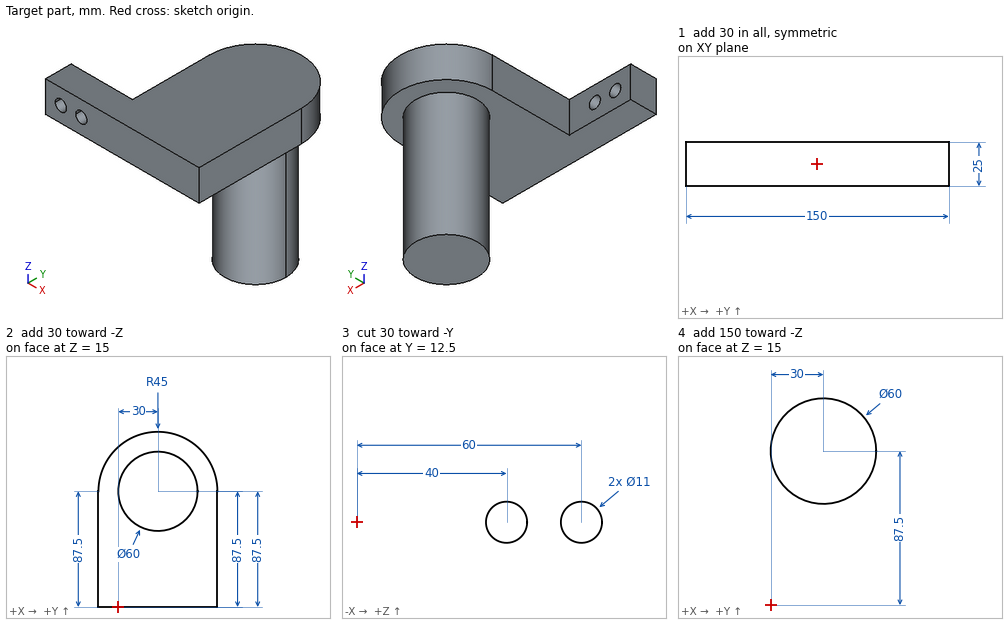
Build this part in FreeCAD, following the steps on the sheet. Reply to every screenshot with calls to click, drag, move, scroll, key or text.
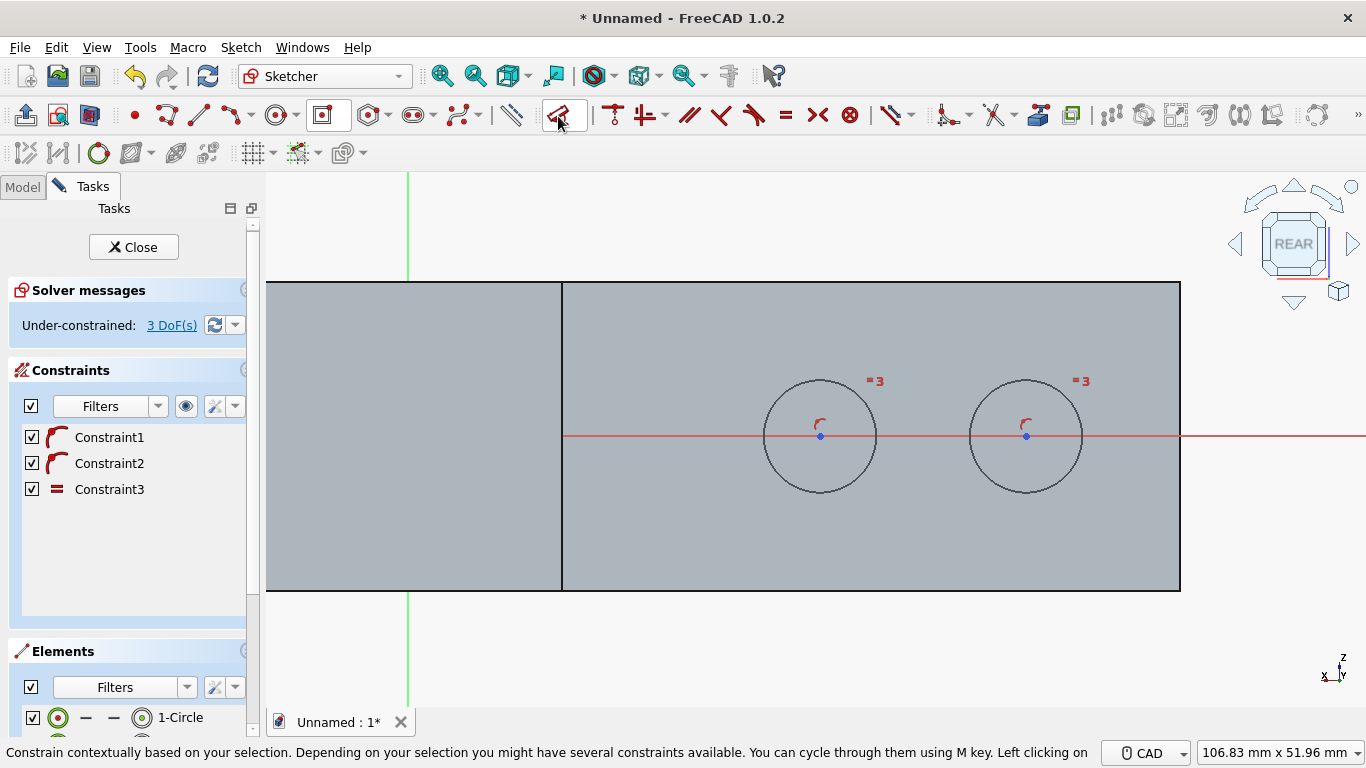
click(1066, 397)
click(1089, 375)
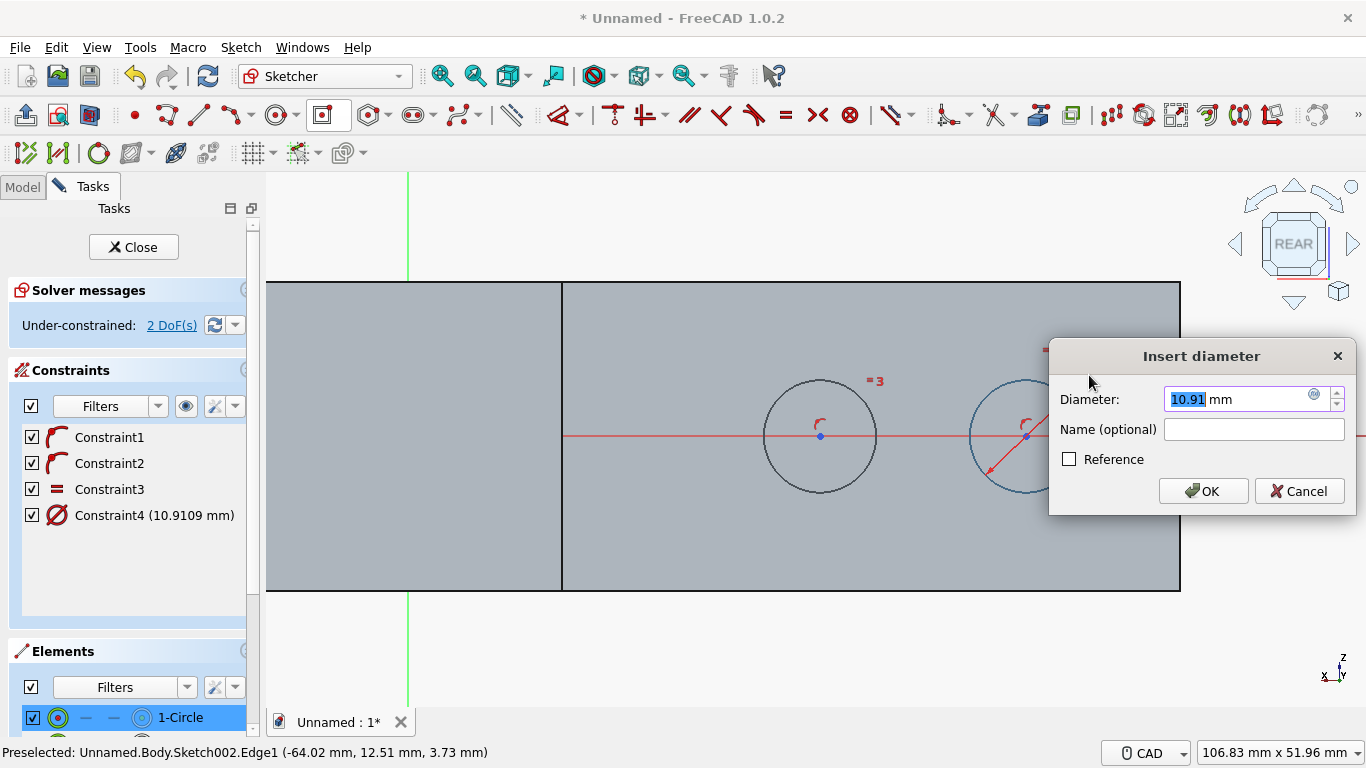
text(11)
key(Return)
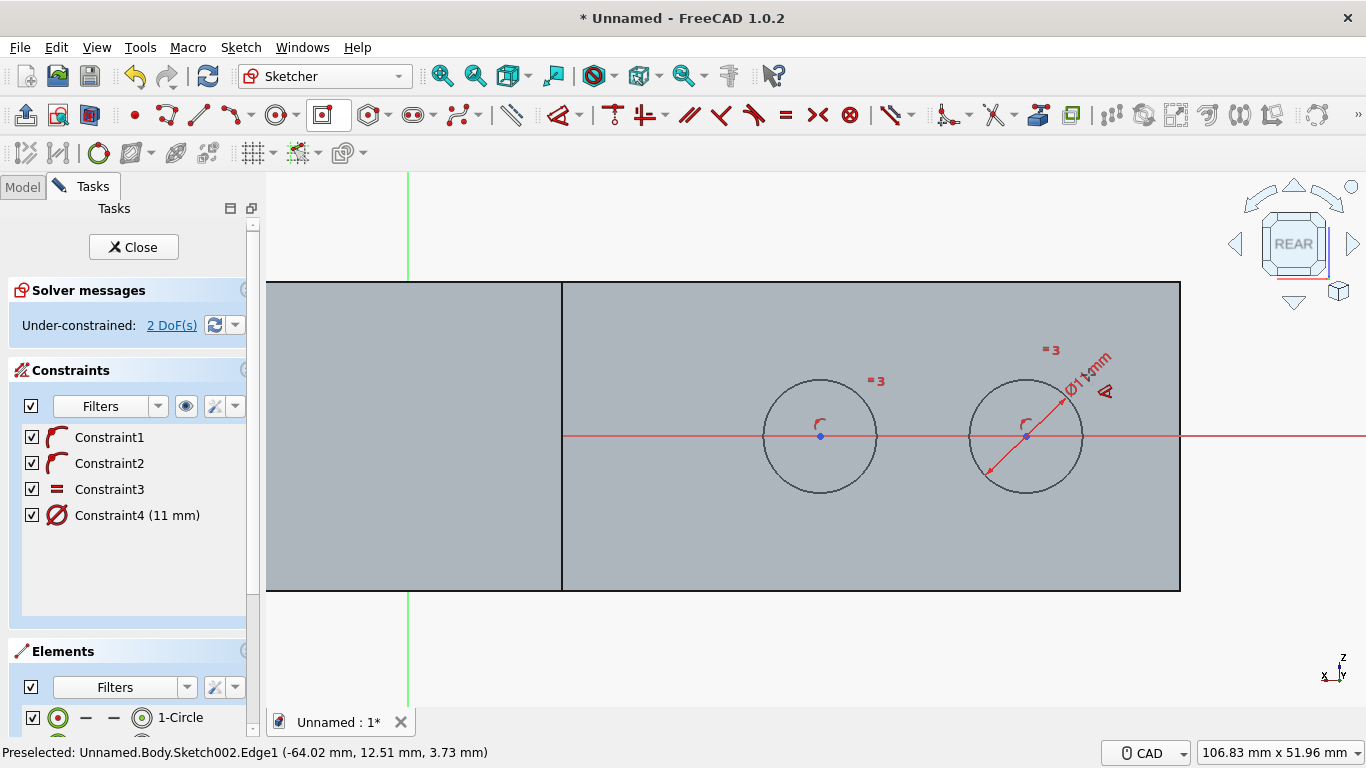
click(1026, 436)
click(717, 470)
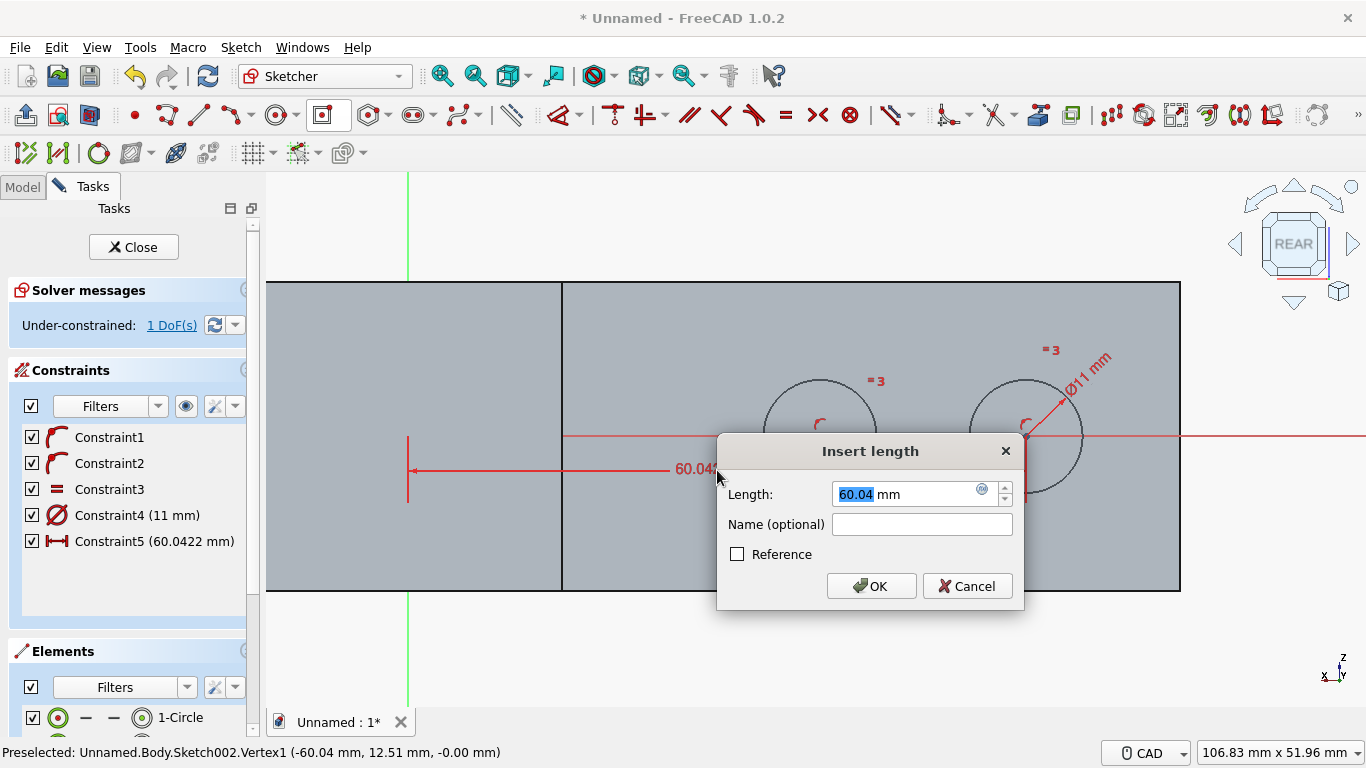
text(60)
key(Return)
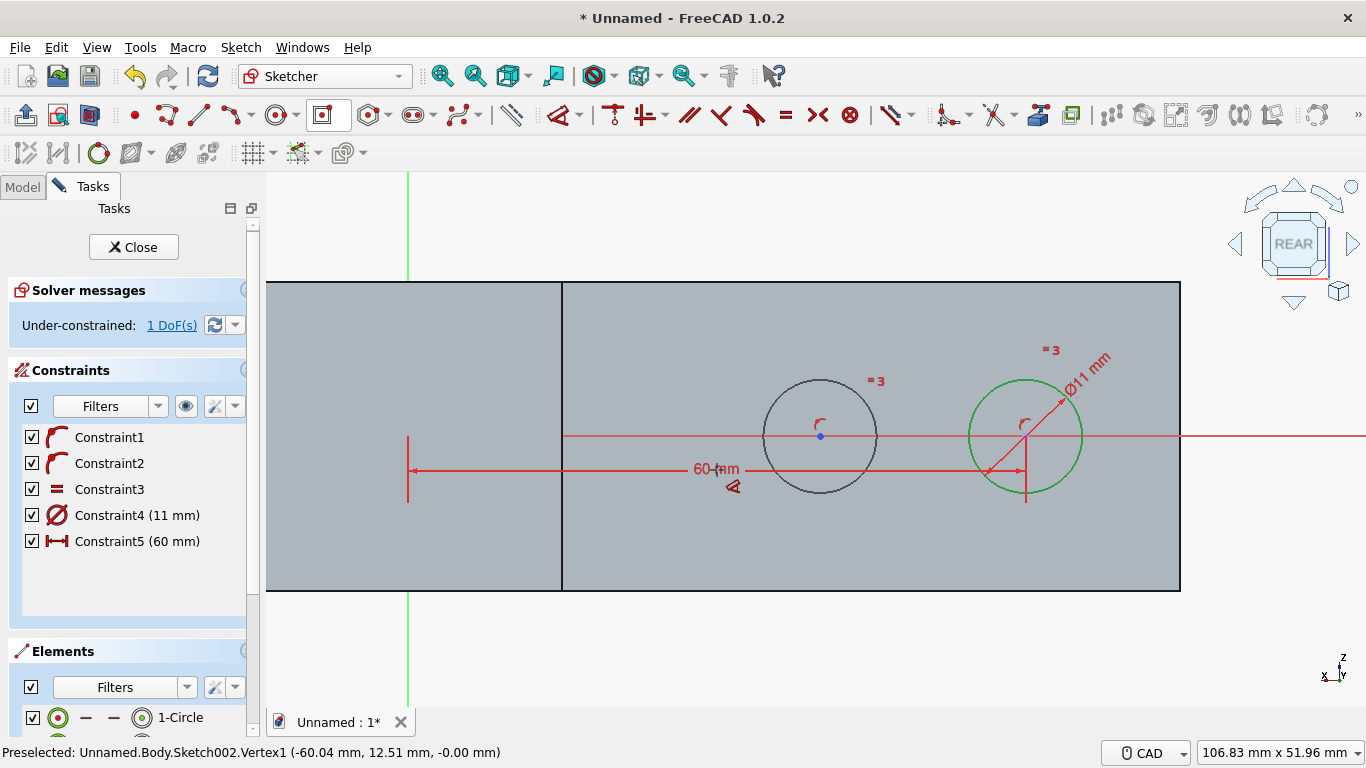
click(820, 436)
click(614, 470)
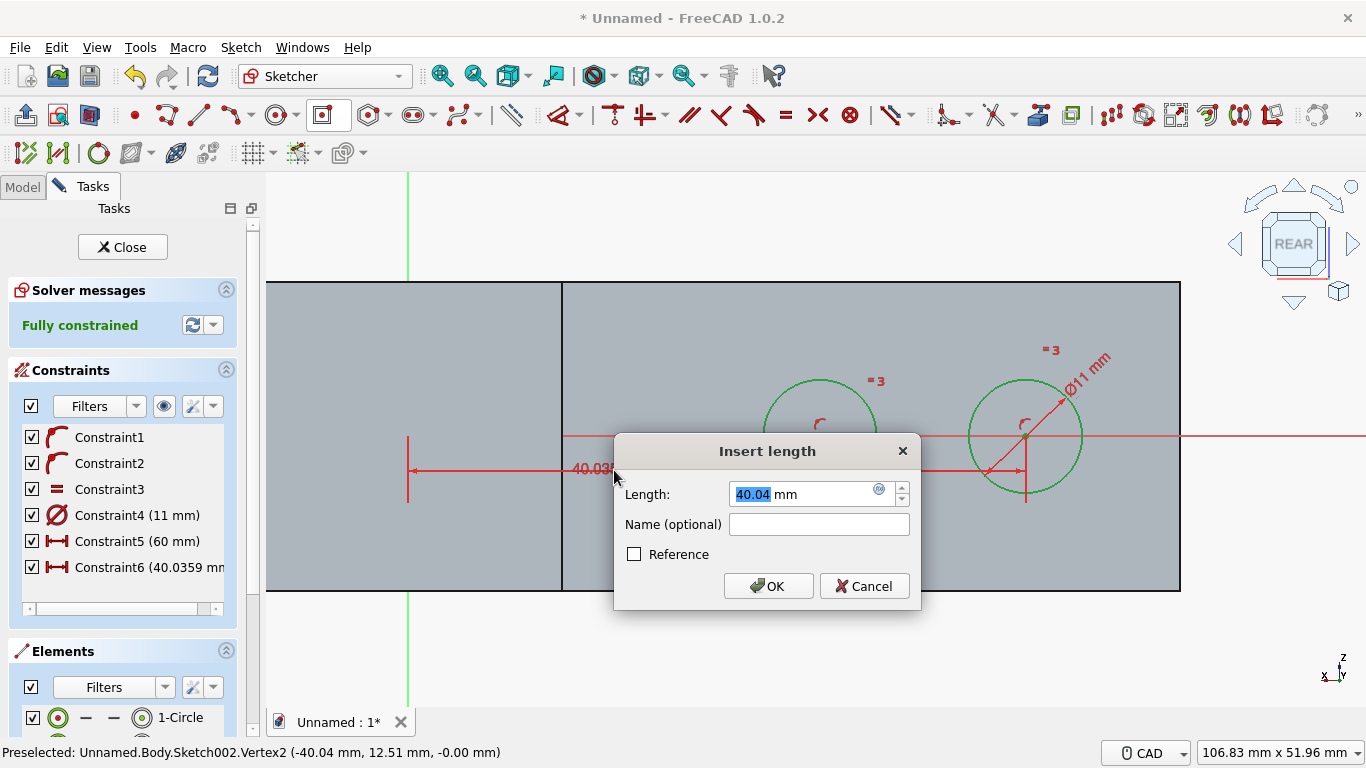
text(40)
key(Return)
key(Escape)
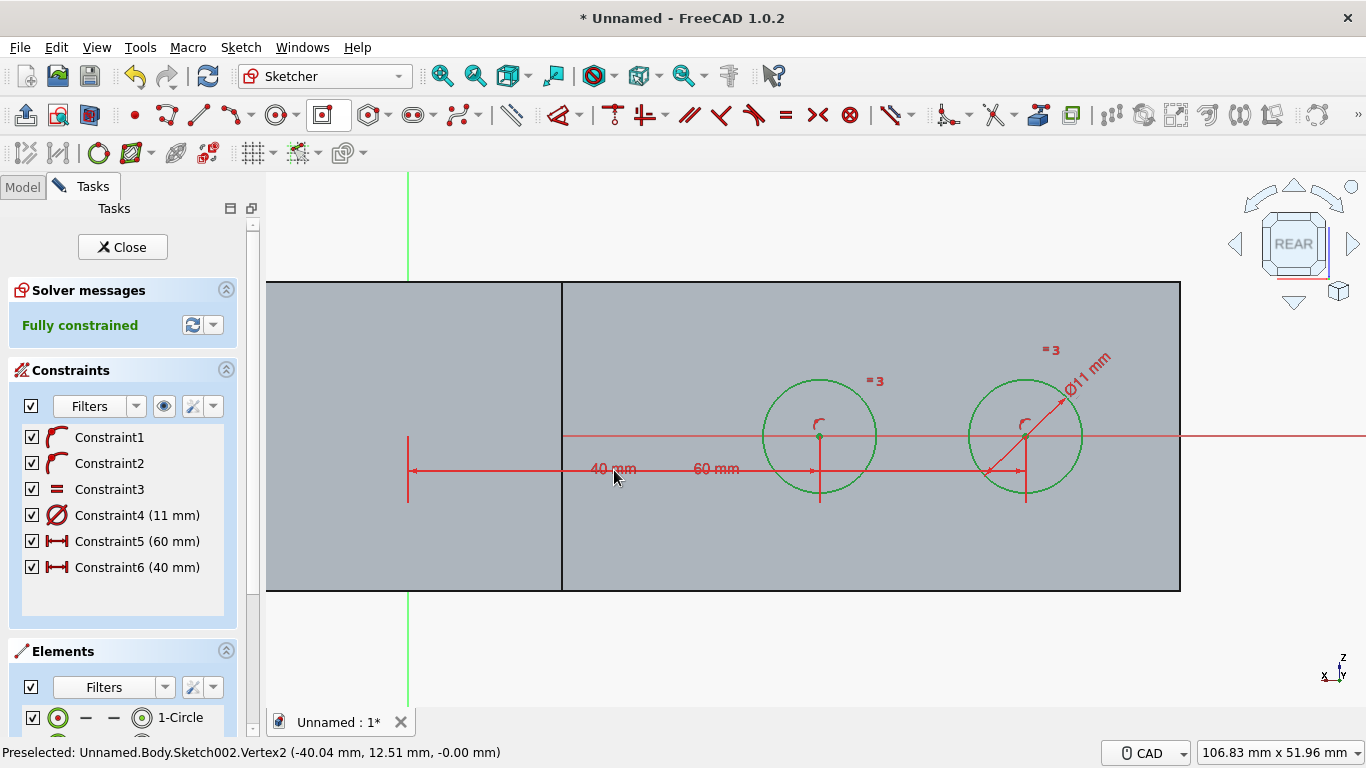
click(123, 247)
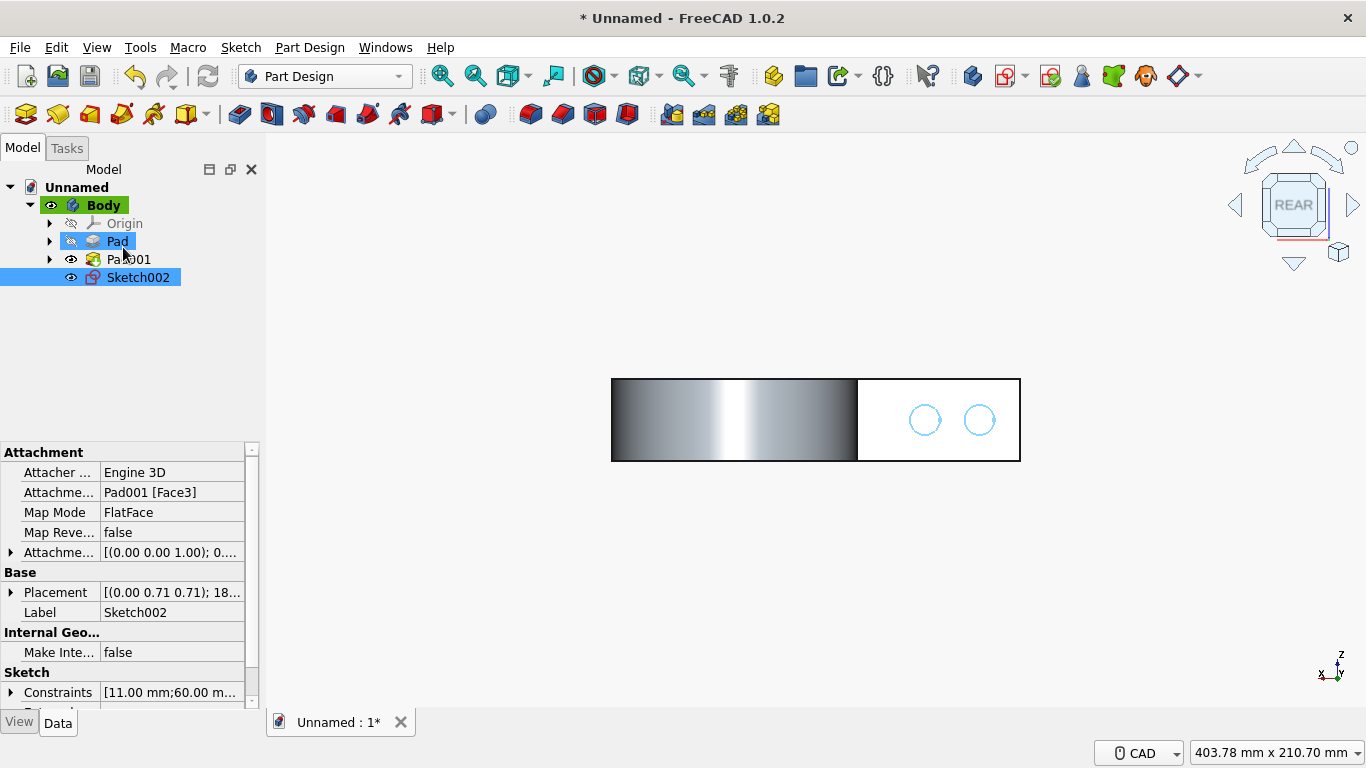
click(240, 114)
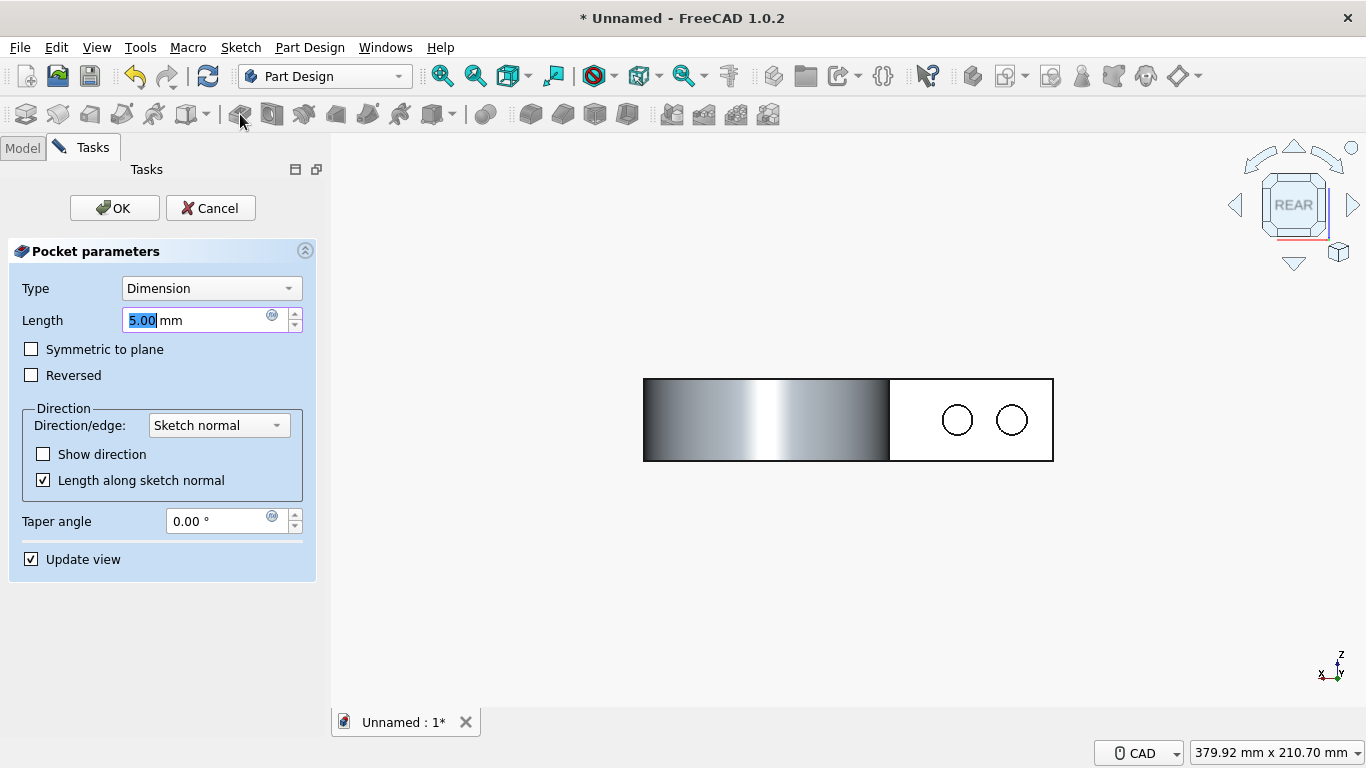
text(30)
key(Tab)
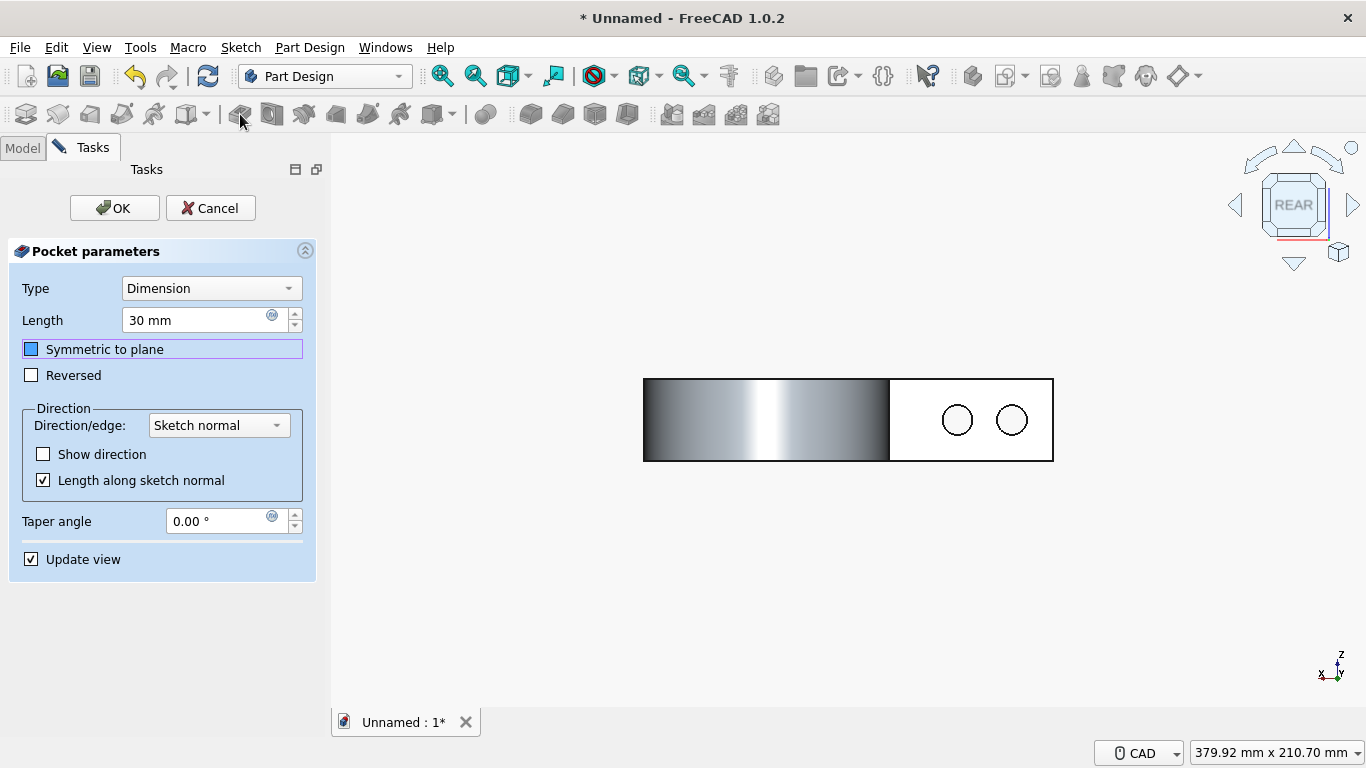
click(115, 208)